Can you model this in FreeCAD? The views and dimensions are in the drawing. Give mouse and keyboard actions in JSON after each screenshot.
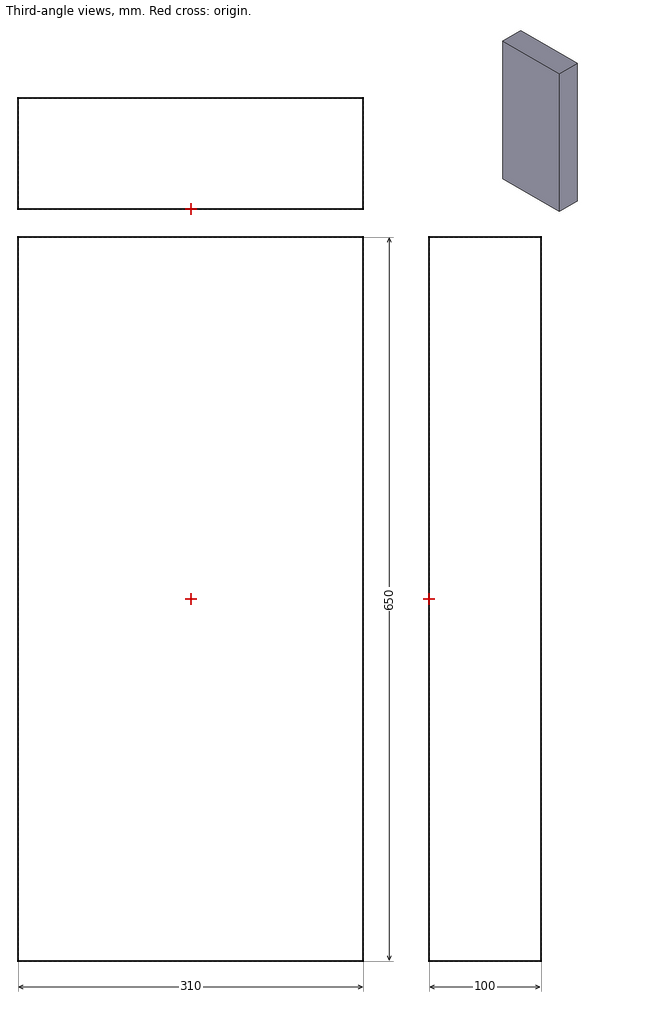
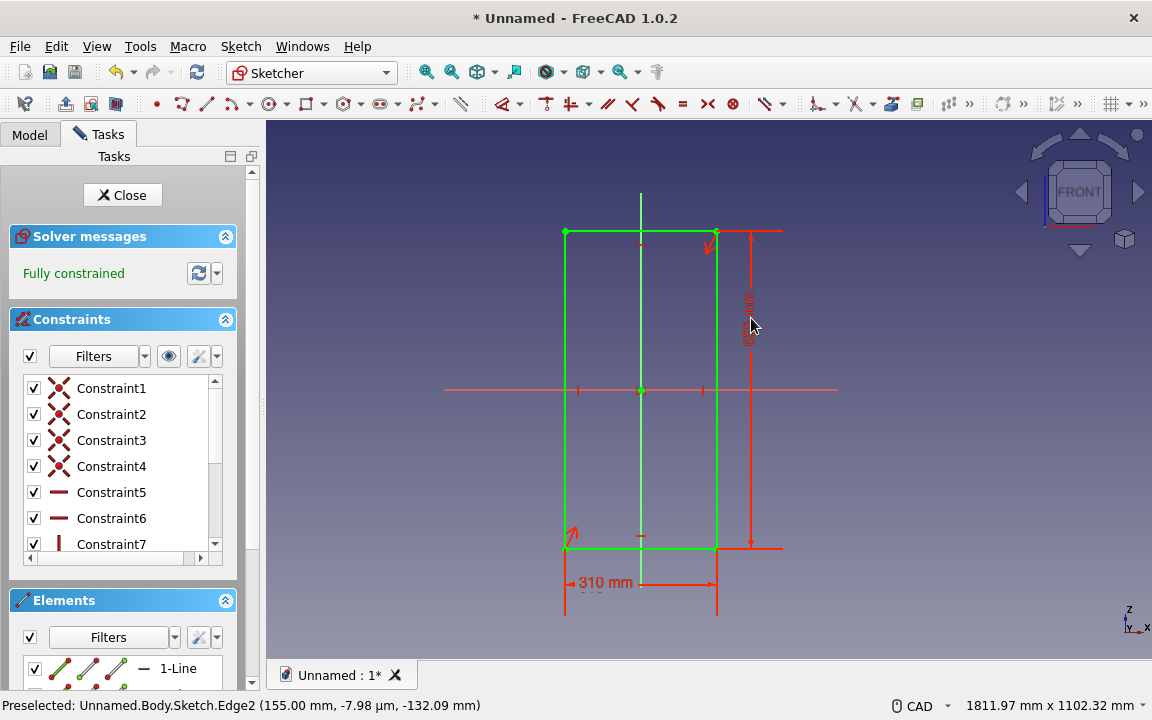
{"action": "left_click", "coordinate": [123, 195]}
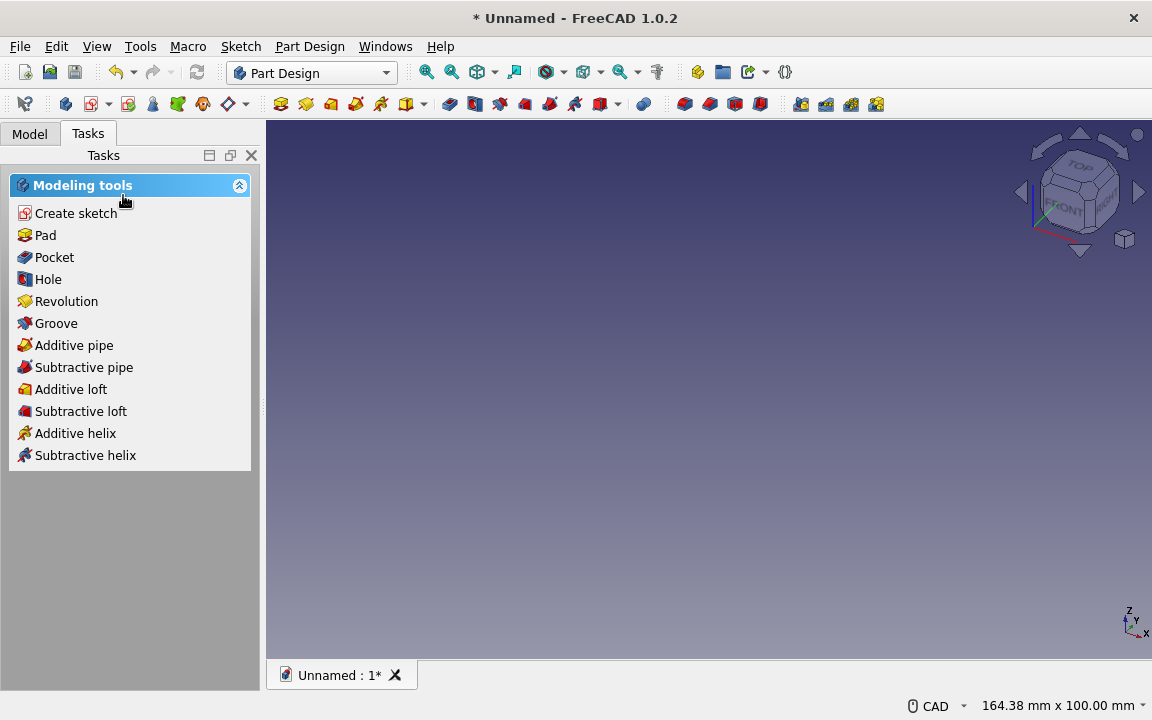
{"action": "left_click", "coordinate": [281, 104]}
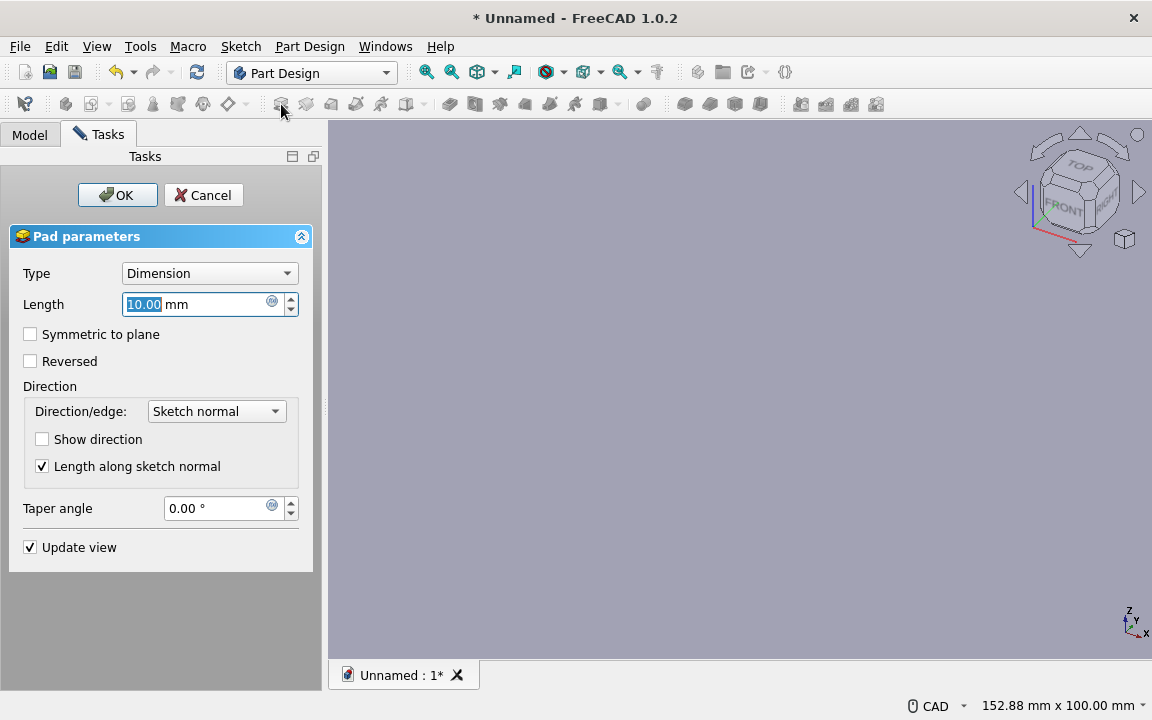
{"action": "type", "text": "100"}
{"action": "key", "text": "Tab"}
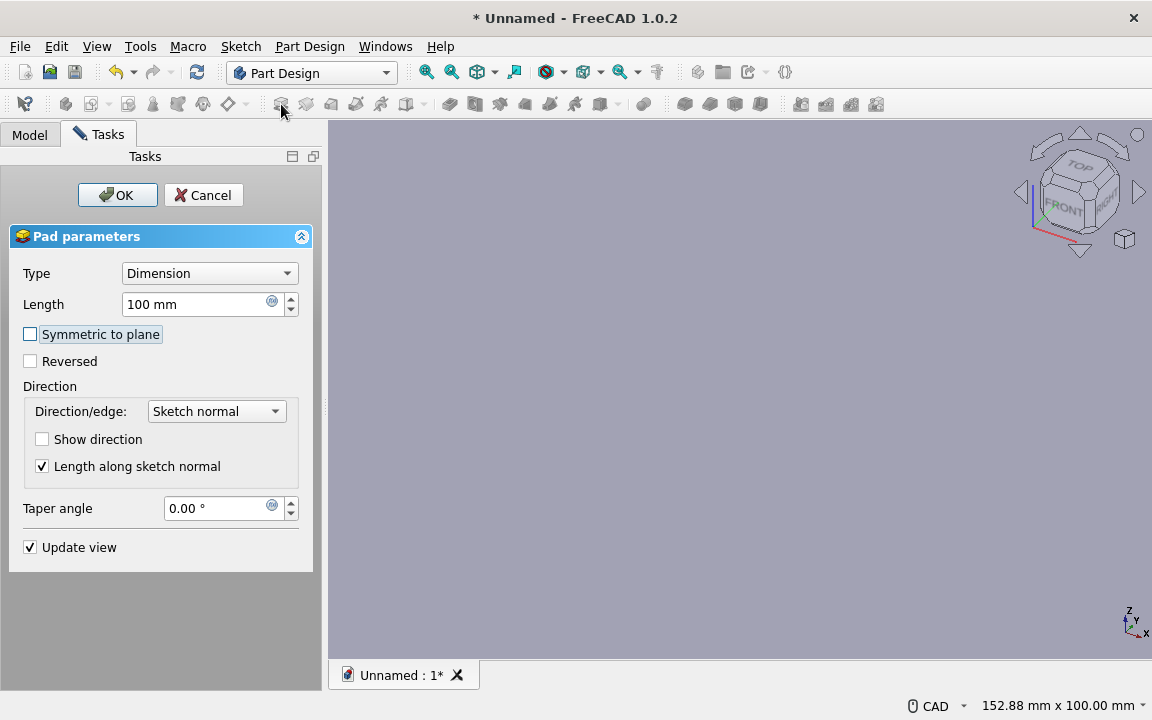
{"action": "left_click", "coordinate": [31, 361]}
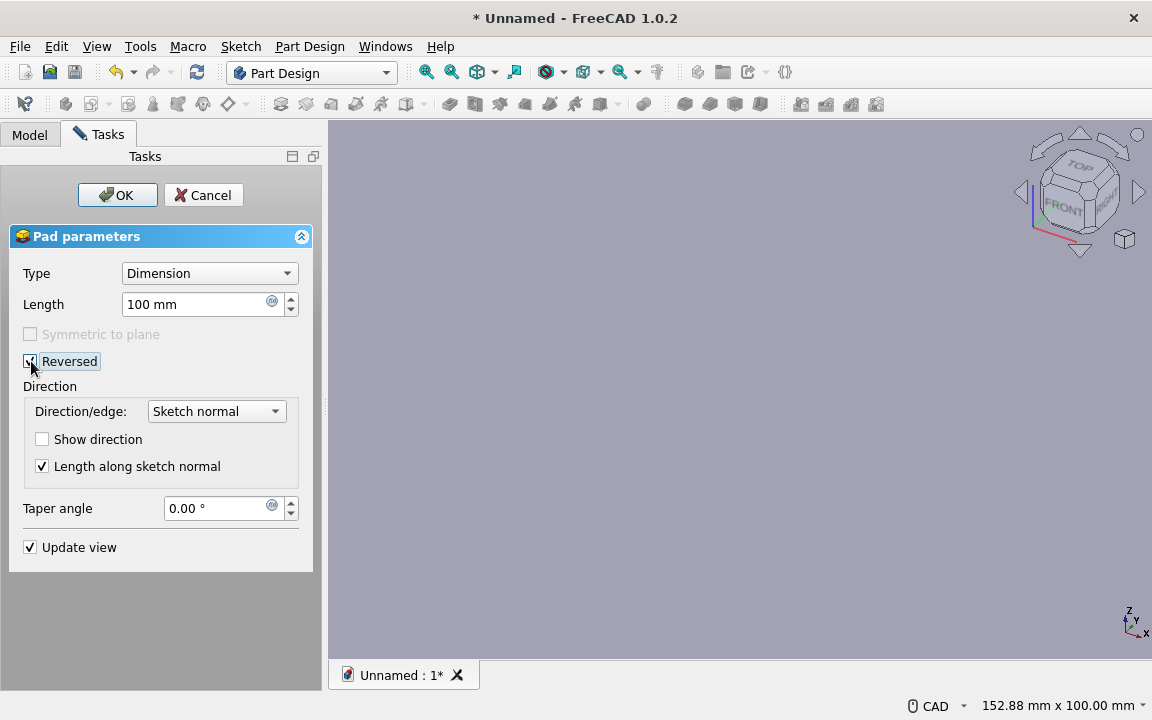
{"action": "left_click", "coordinate": [118, 195]}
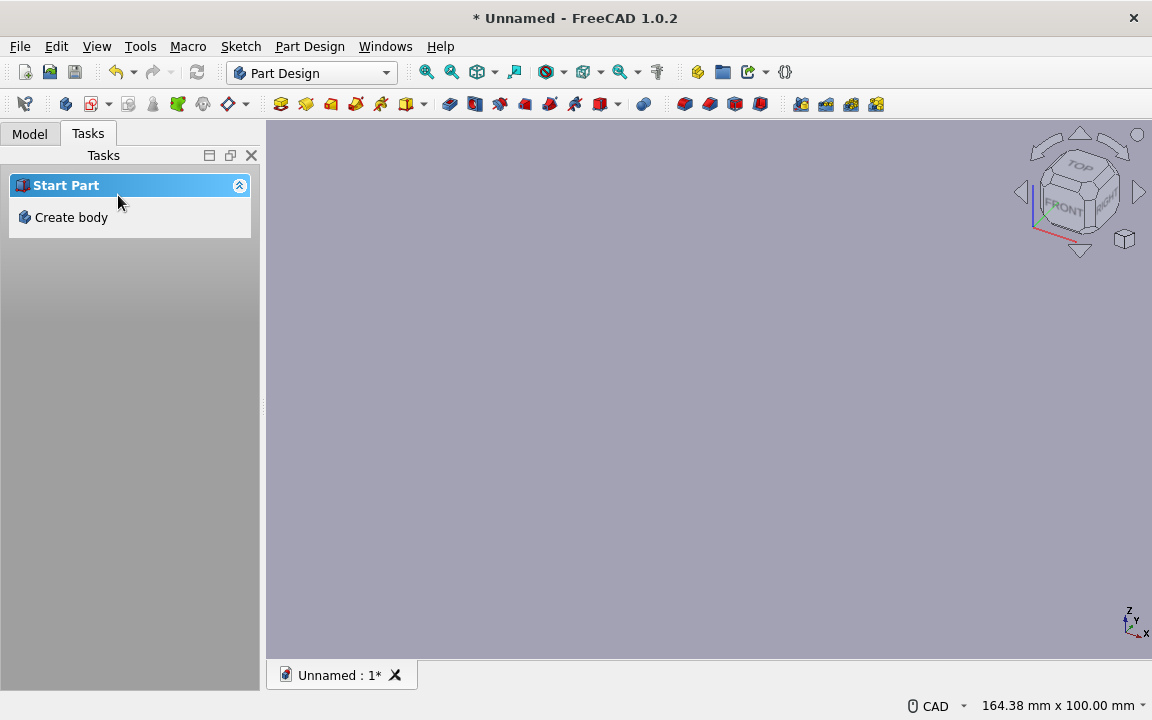
{"action": "key", "text": "0"}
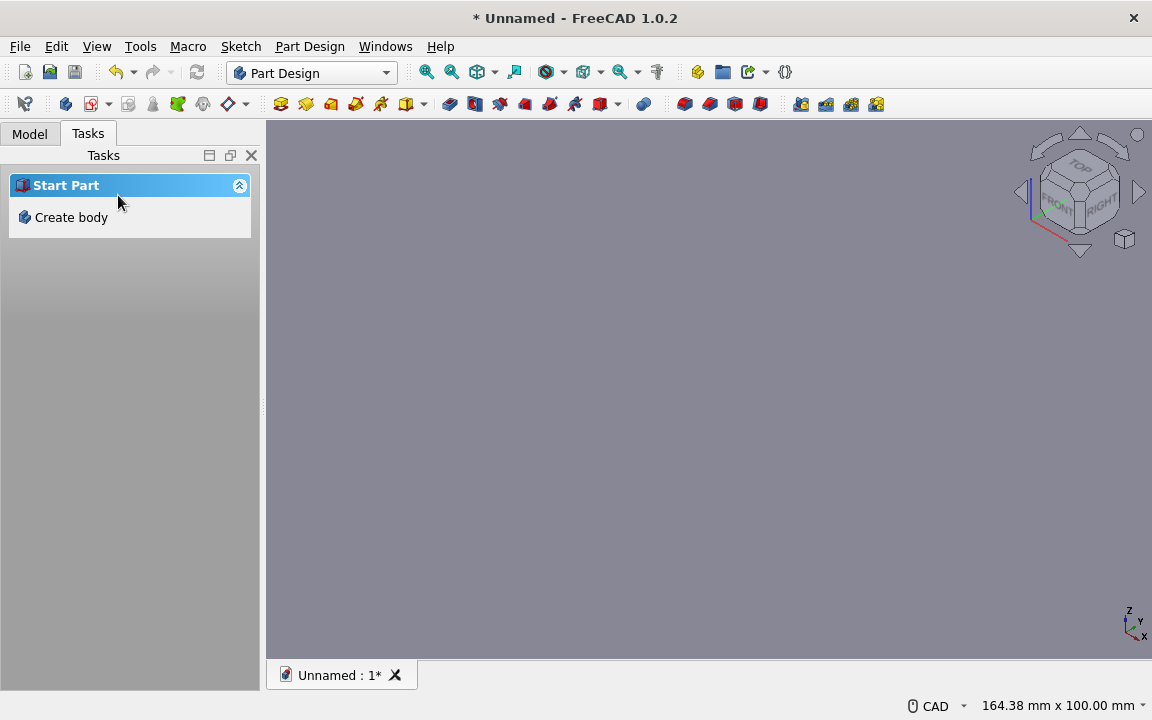
{"action": "left_click", "coordinate": [427, 72]}